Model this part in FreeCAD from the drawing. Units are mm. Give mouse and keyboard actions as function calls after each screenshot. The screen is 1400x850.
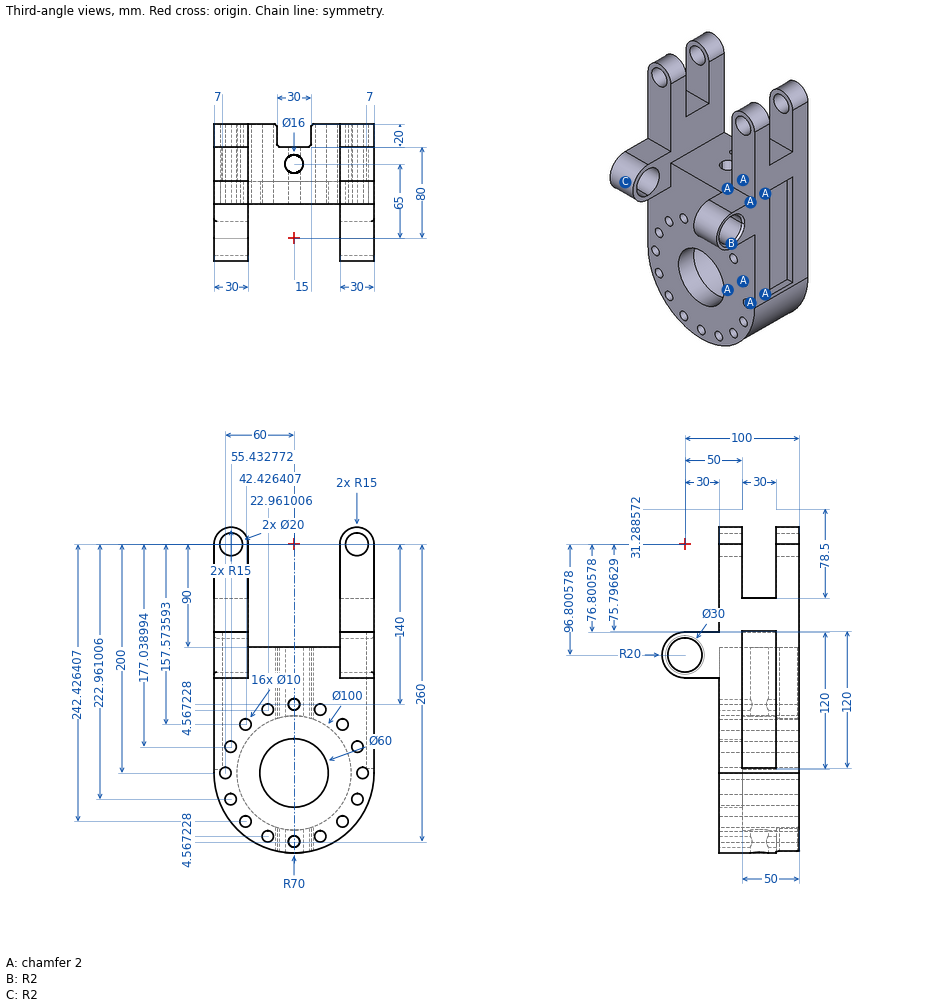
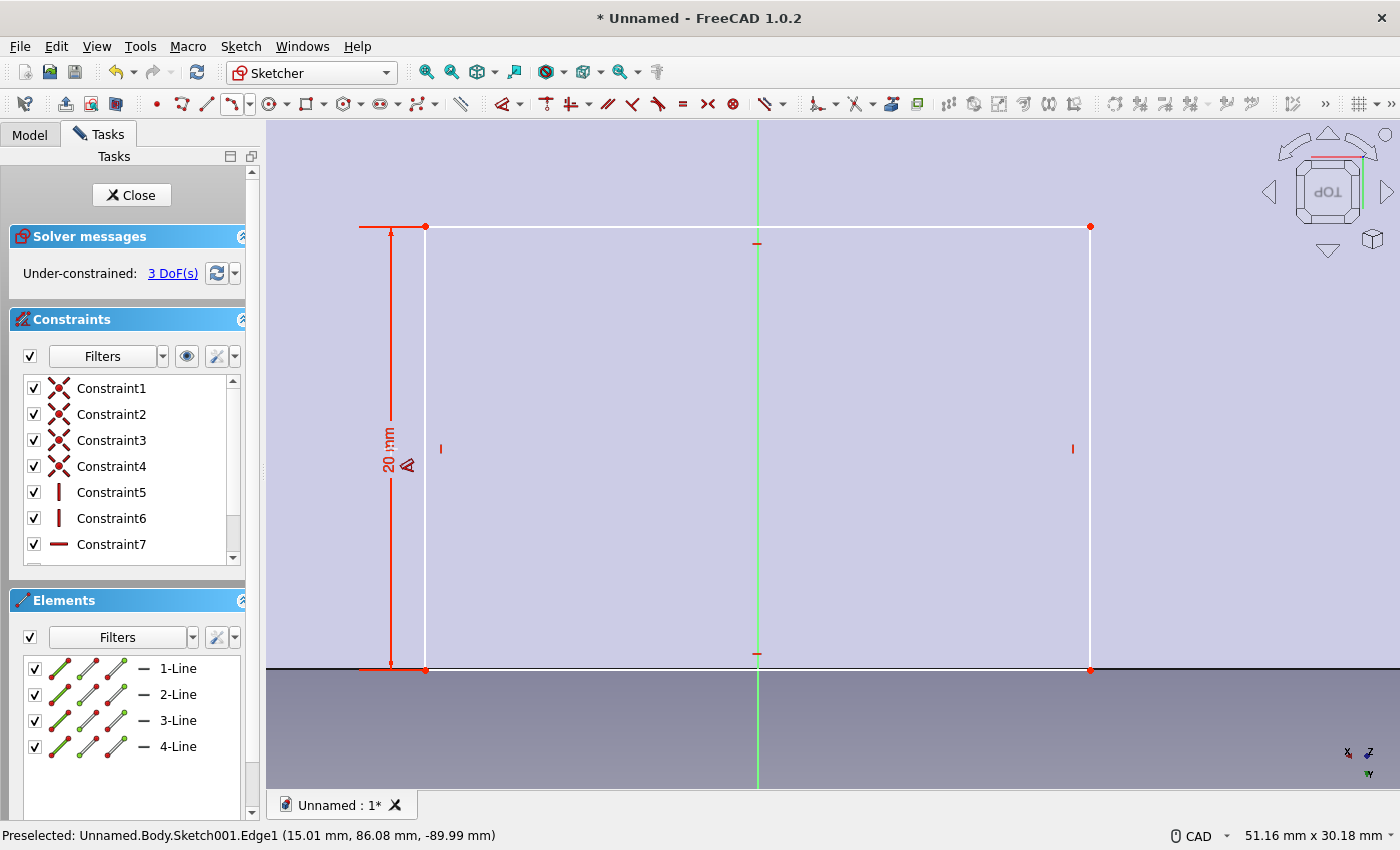
click(625, 670)
click(605, 704)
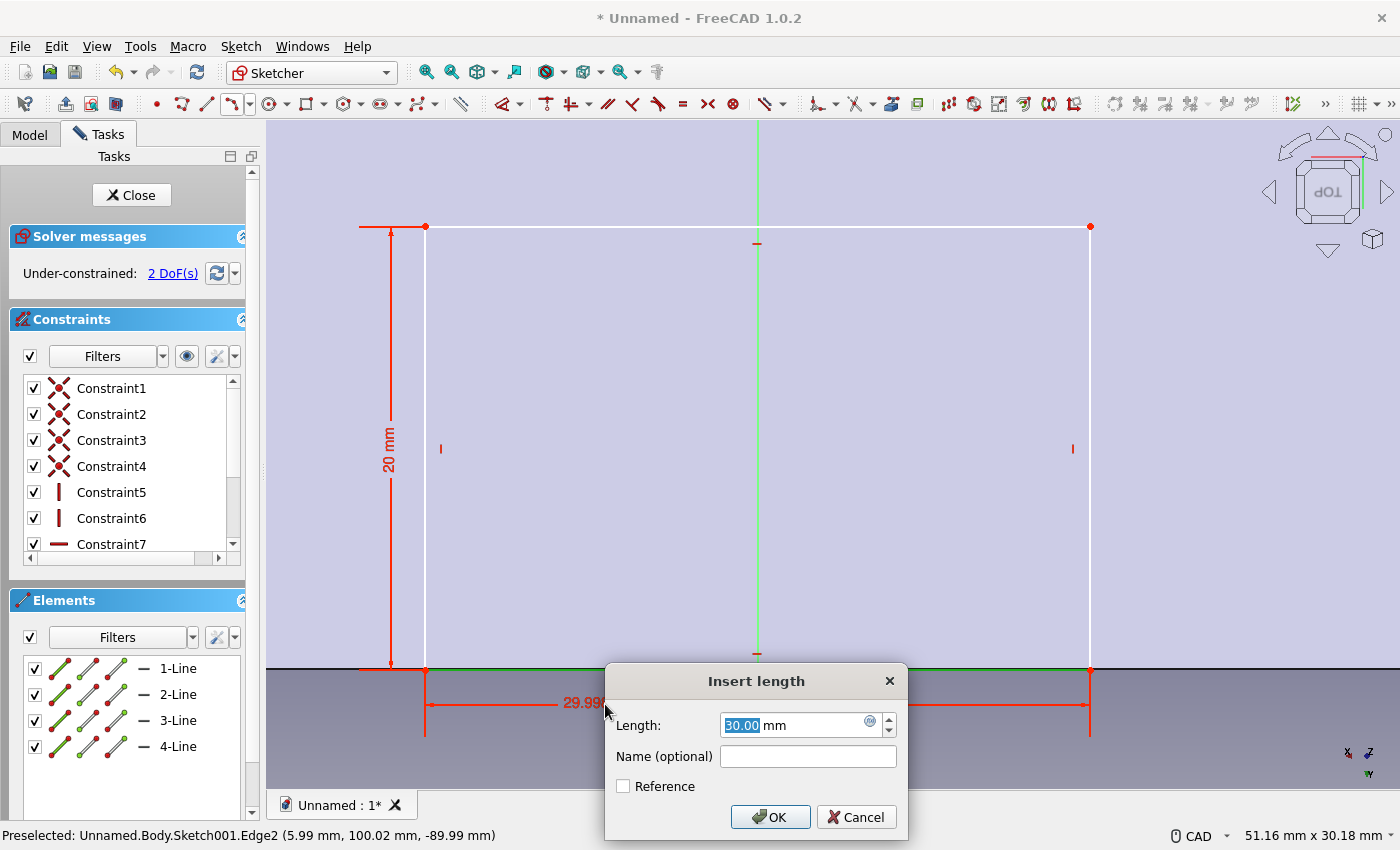
text(30)
key(Return)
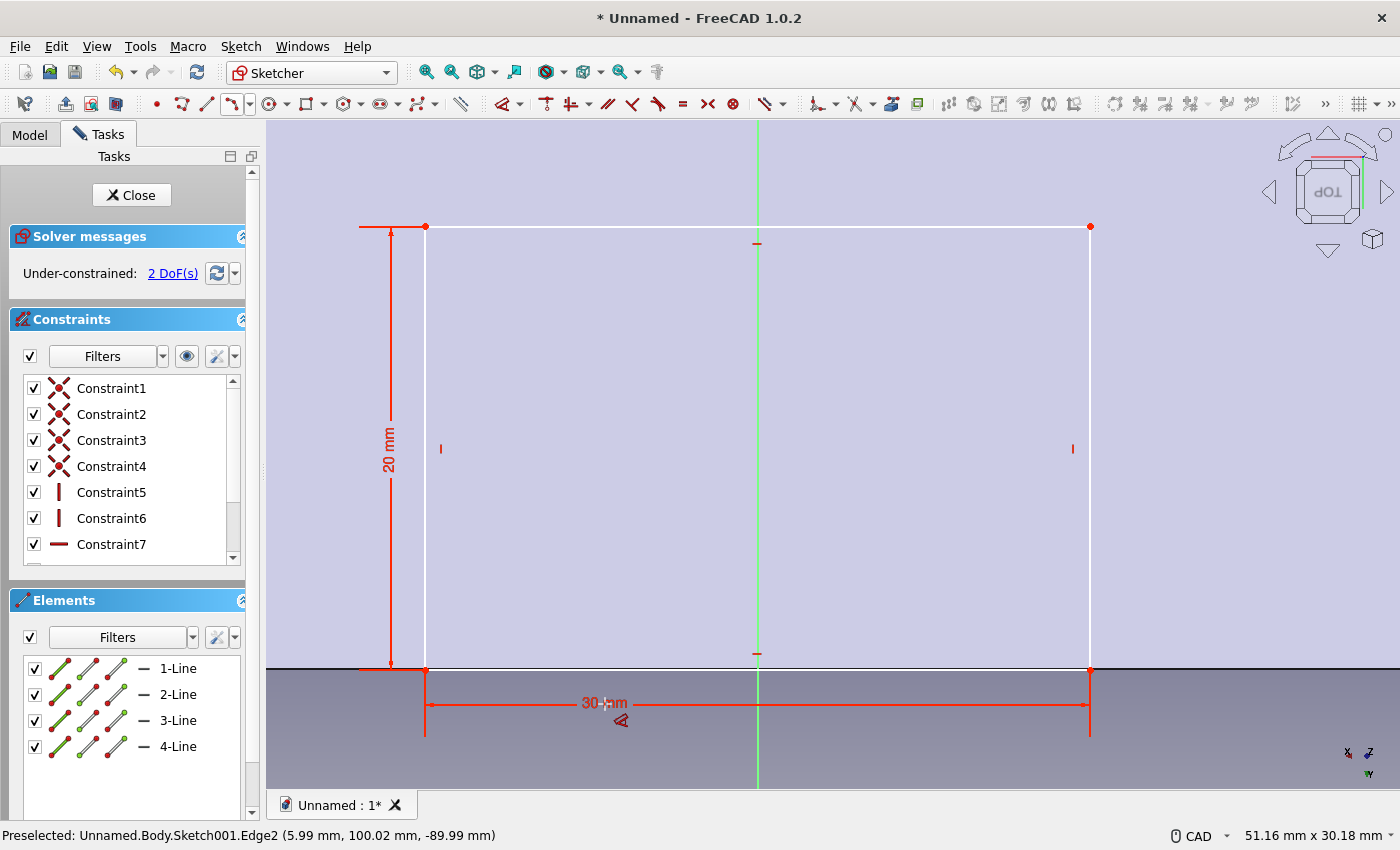
click(425, 227)
click(591, 261)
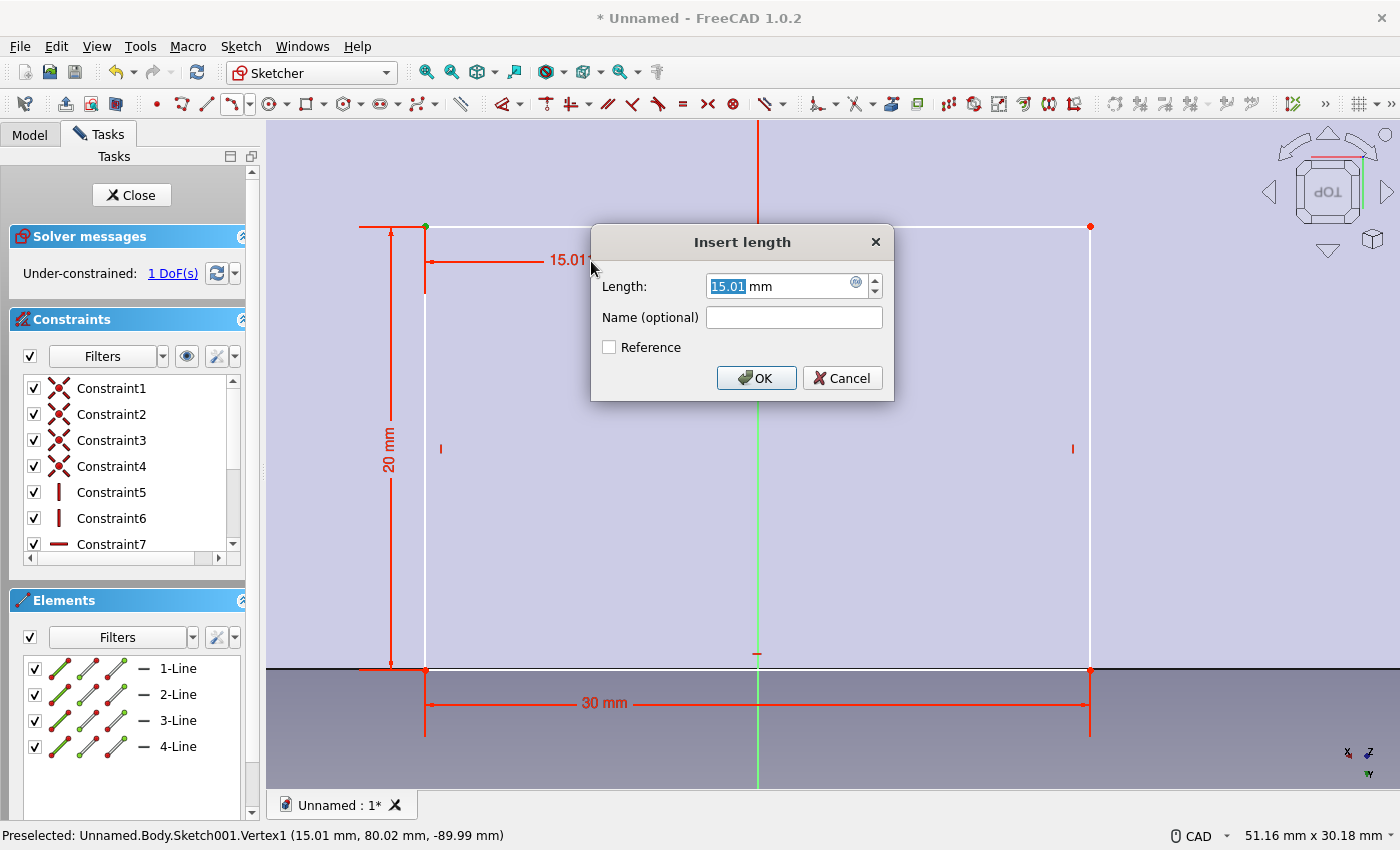
text(15)
key(Return)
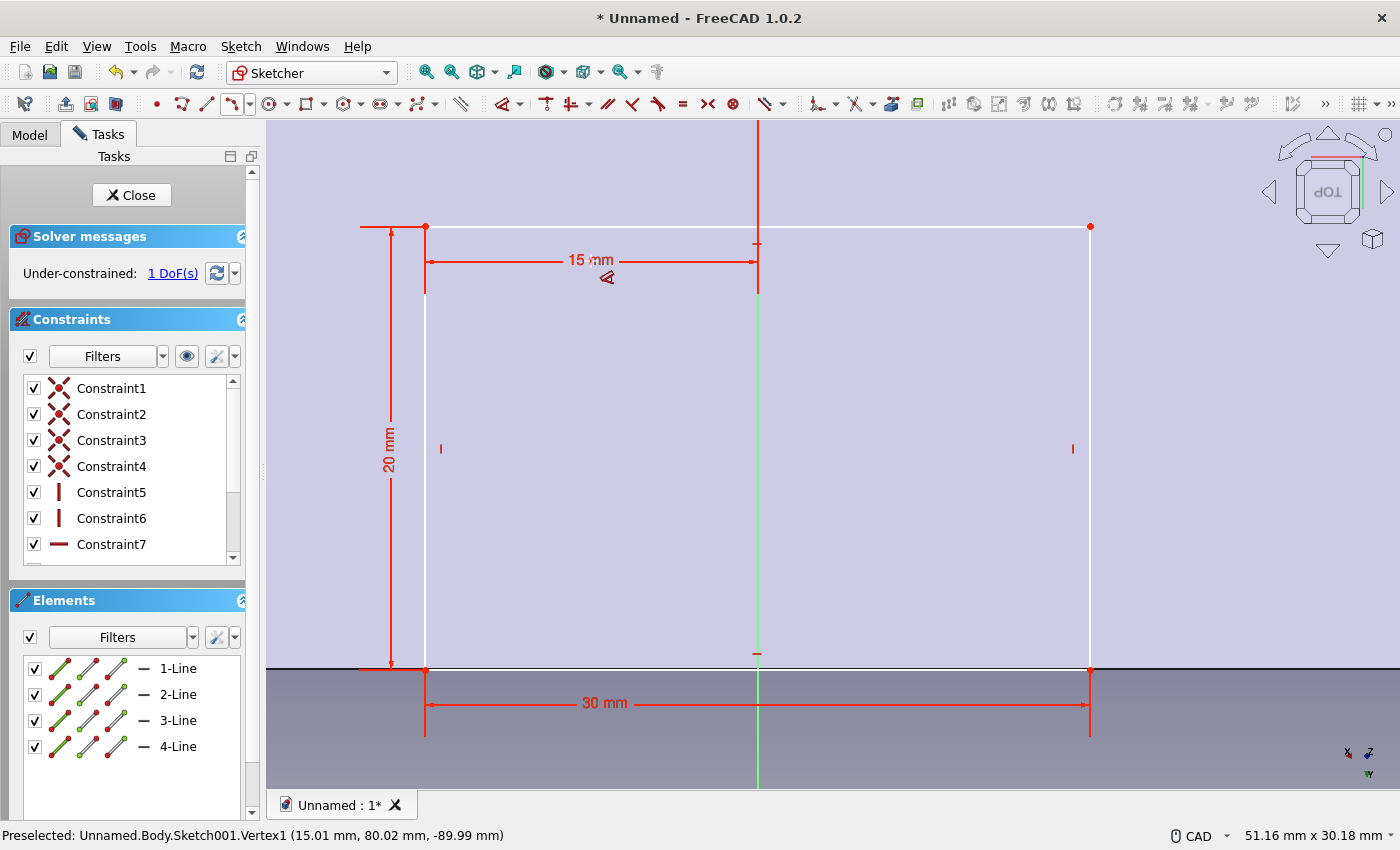
click(425, 227)
click(391, 187)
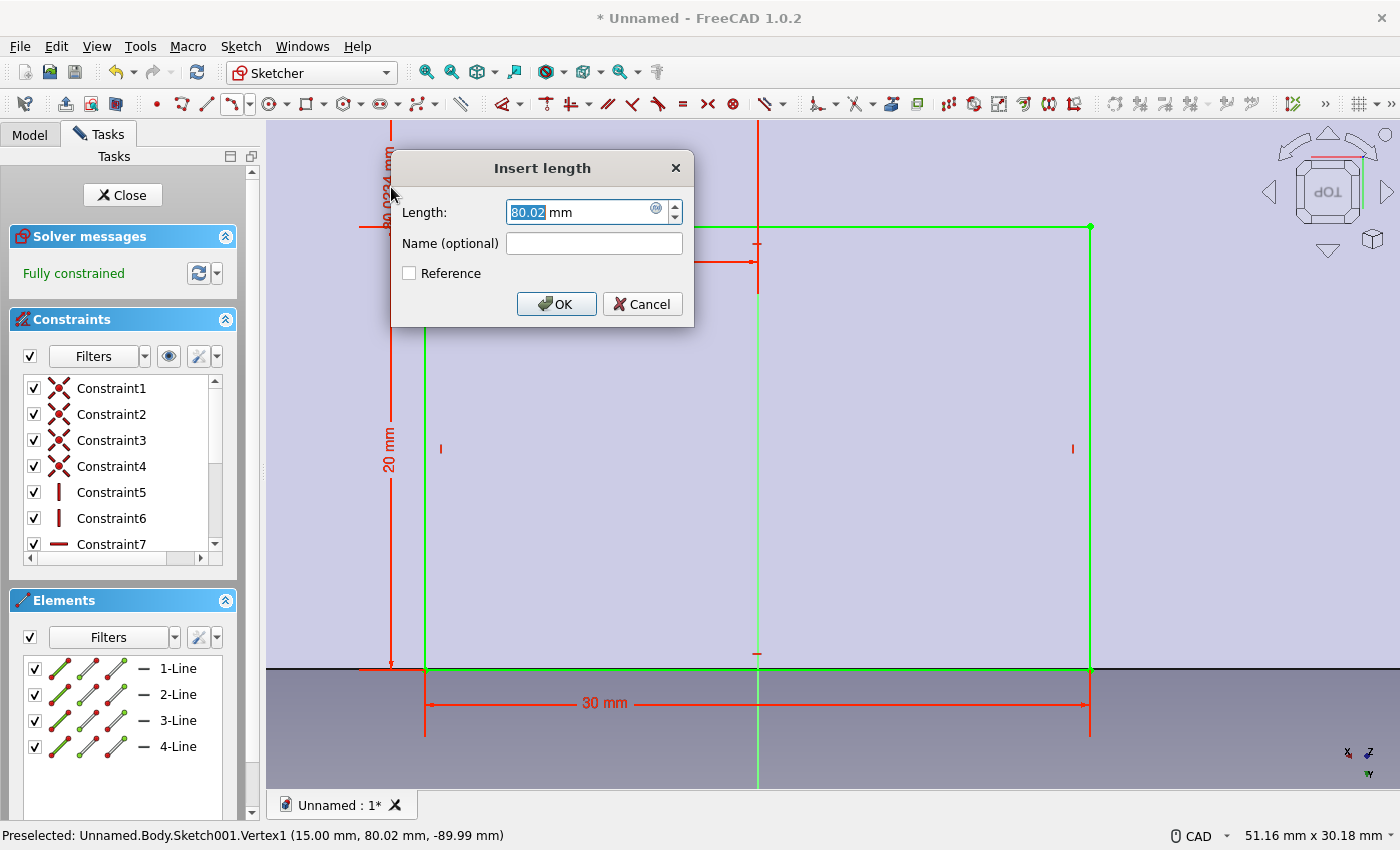
text(80)
key(Return)
key(Escape)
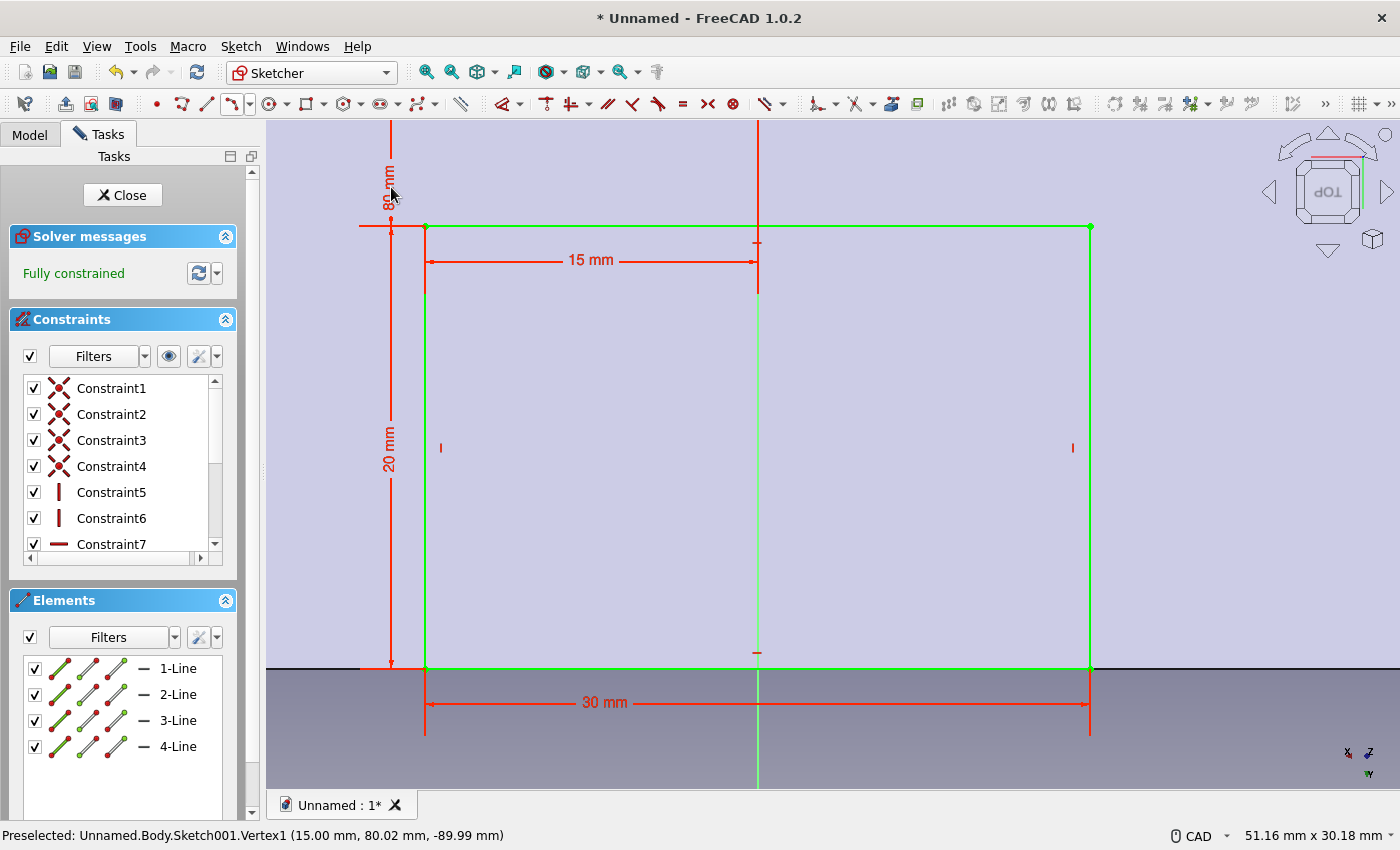
click(123, 195)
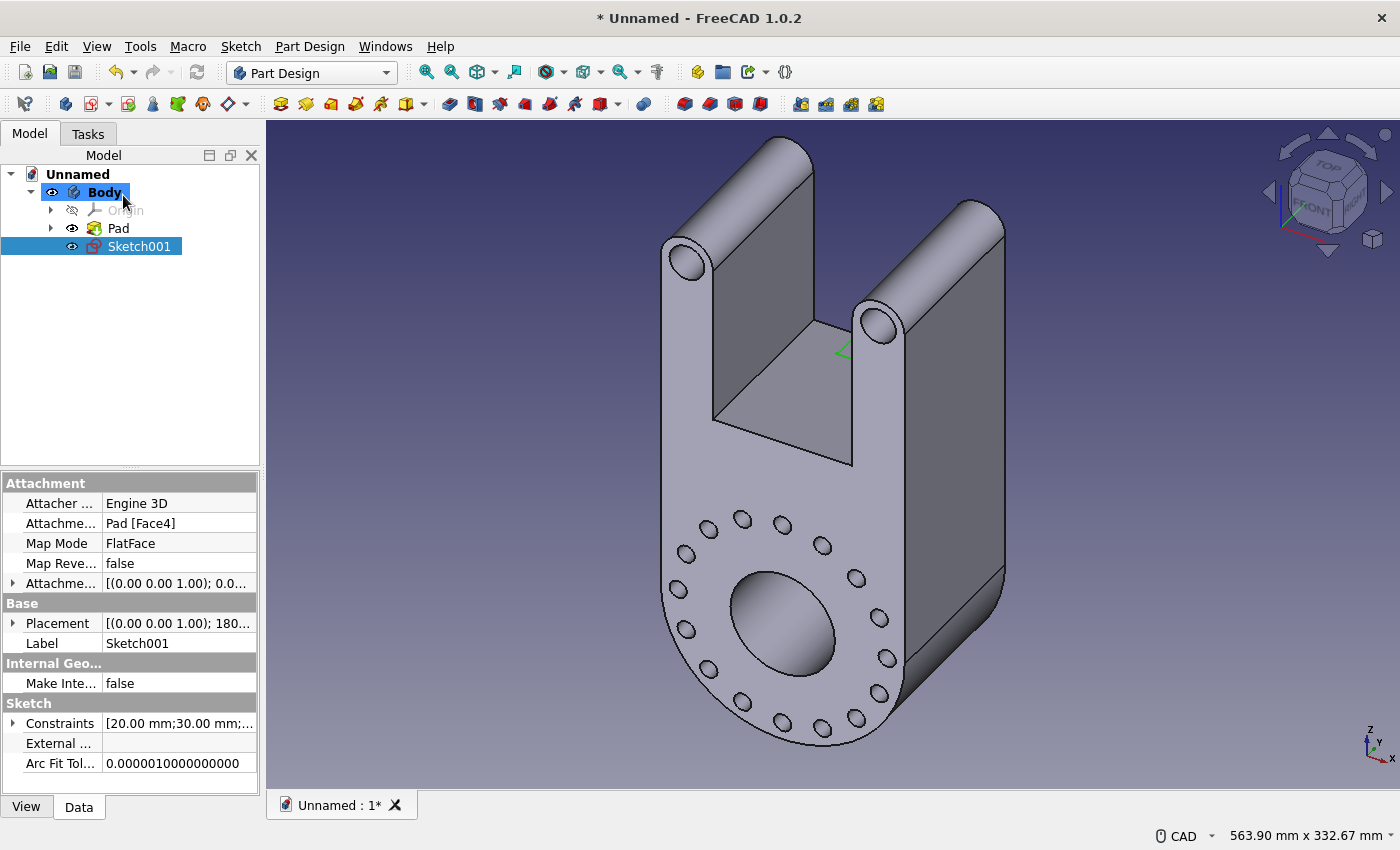
click(450, 104)